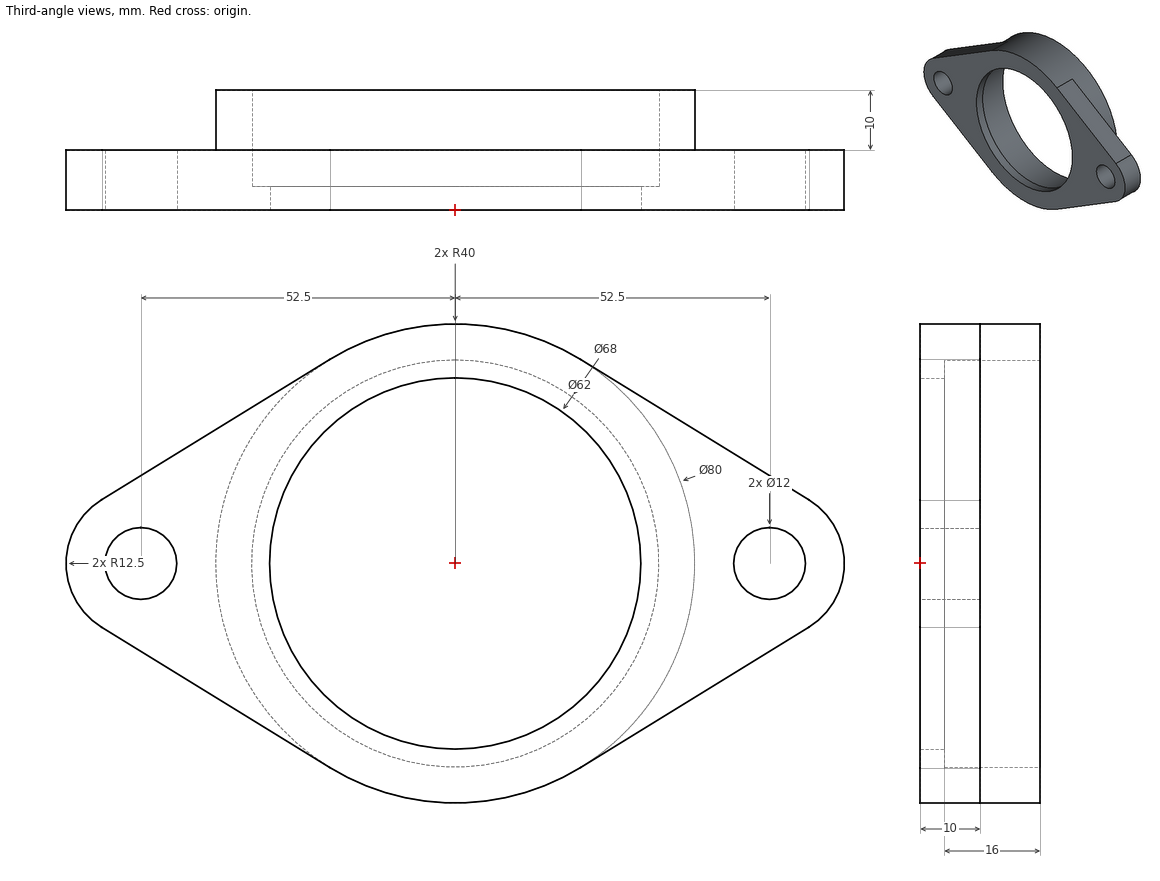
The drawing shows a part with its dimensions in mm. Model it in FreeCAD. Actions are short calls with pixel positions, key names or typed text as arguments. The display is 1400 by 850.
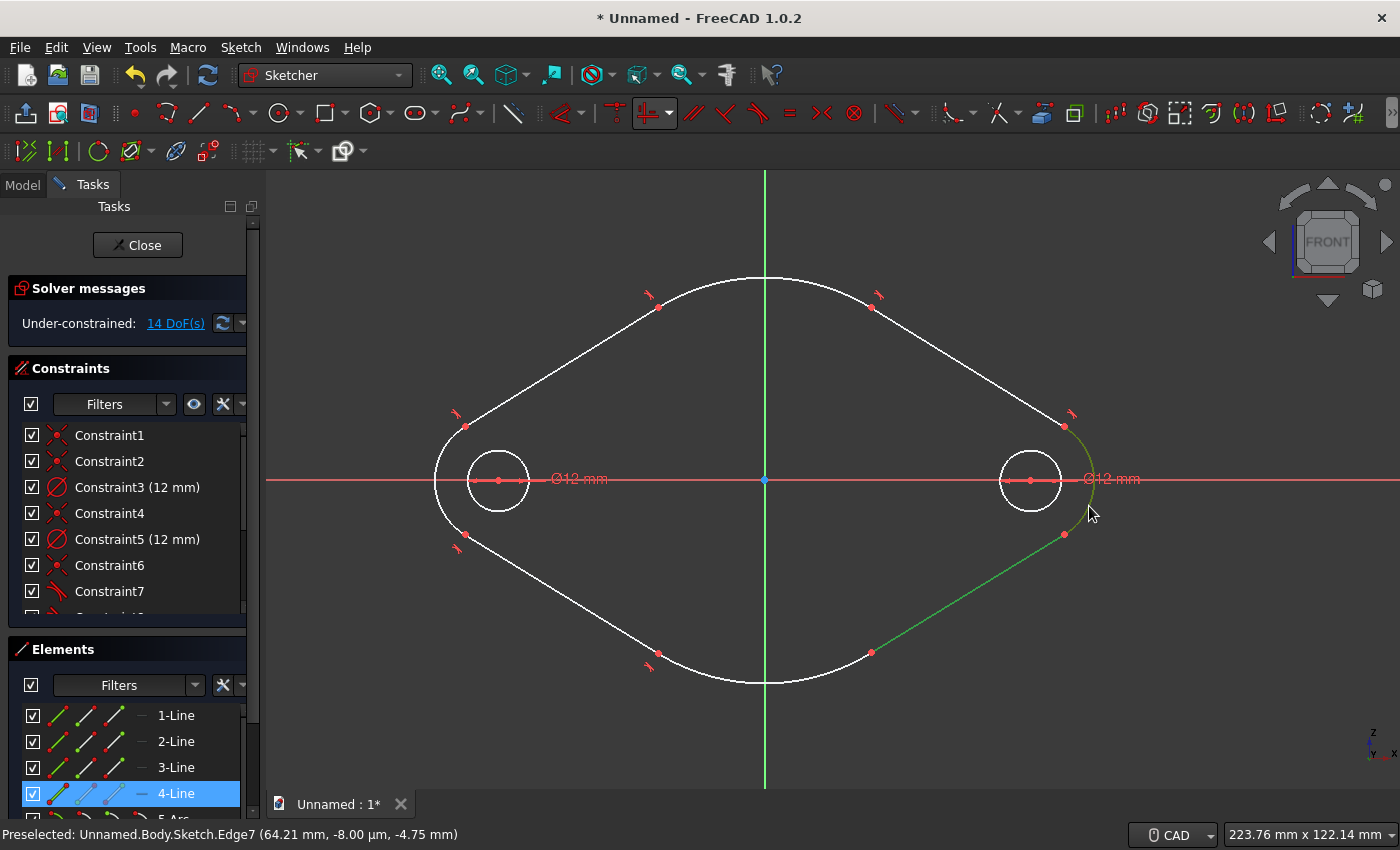
click(758, 114)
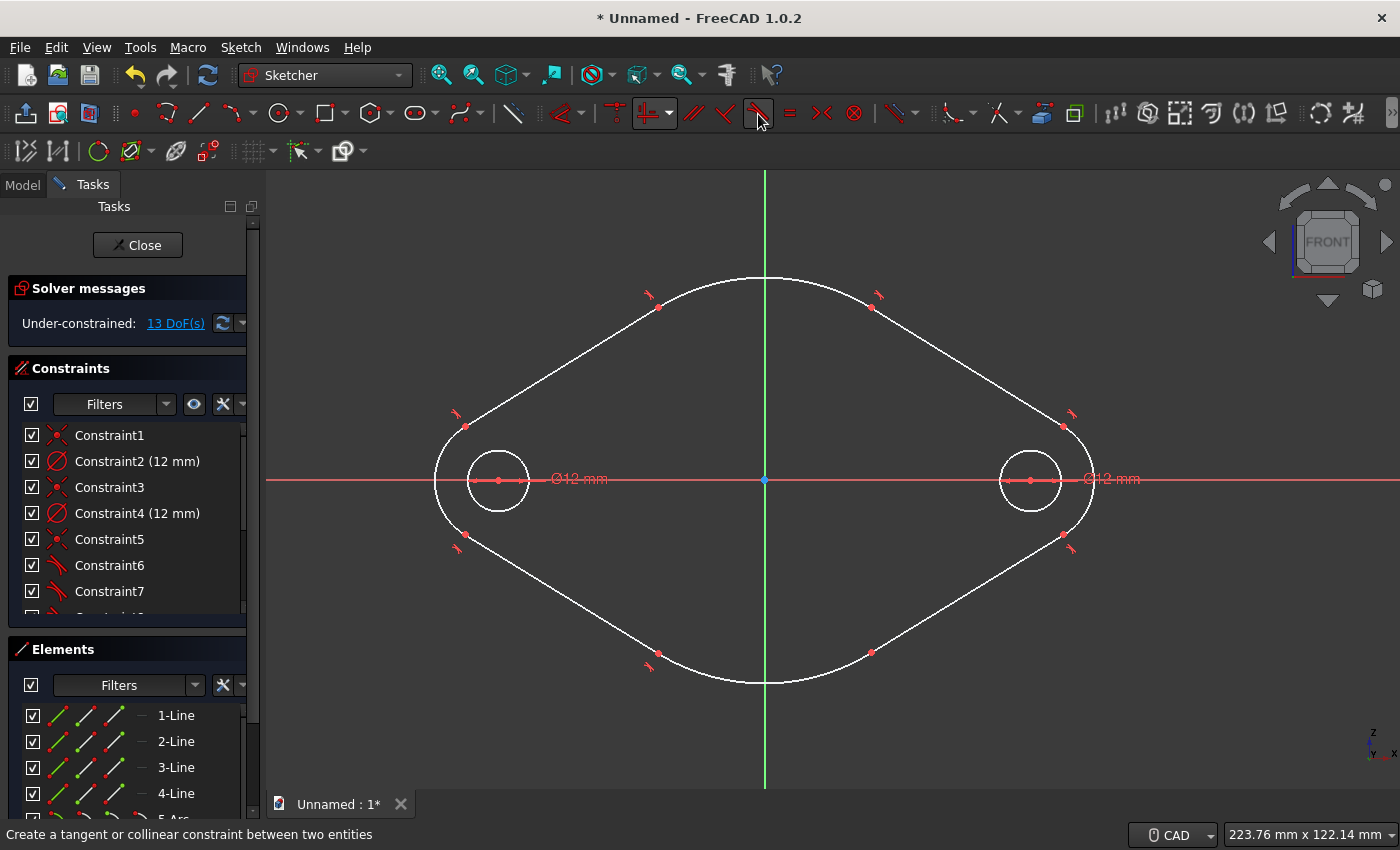
click(1006, 570)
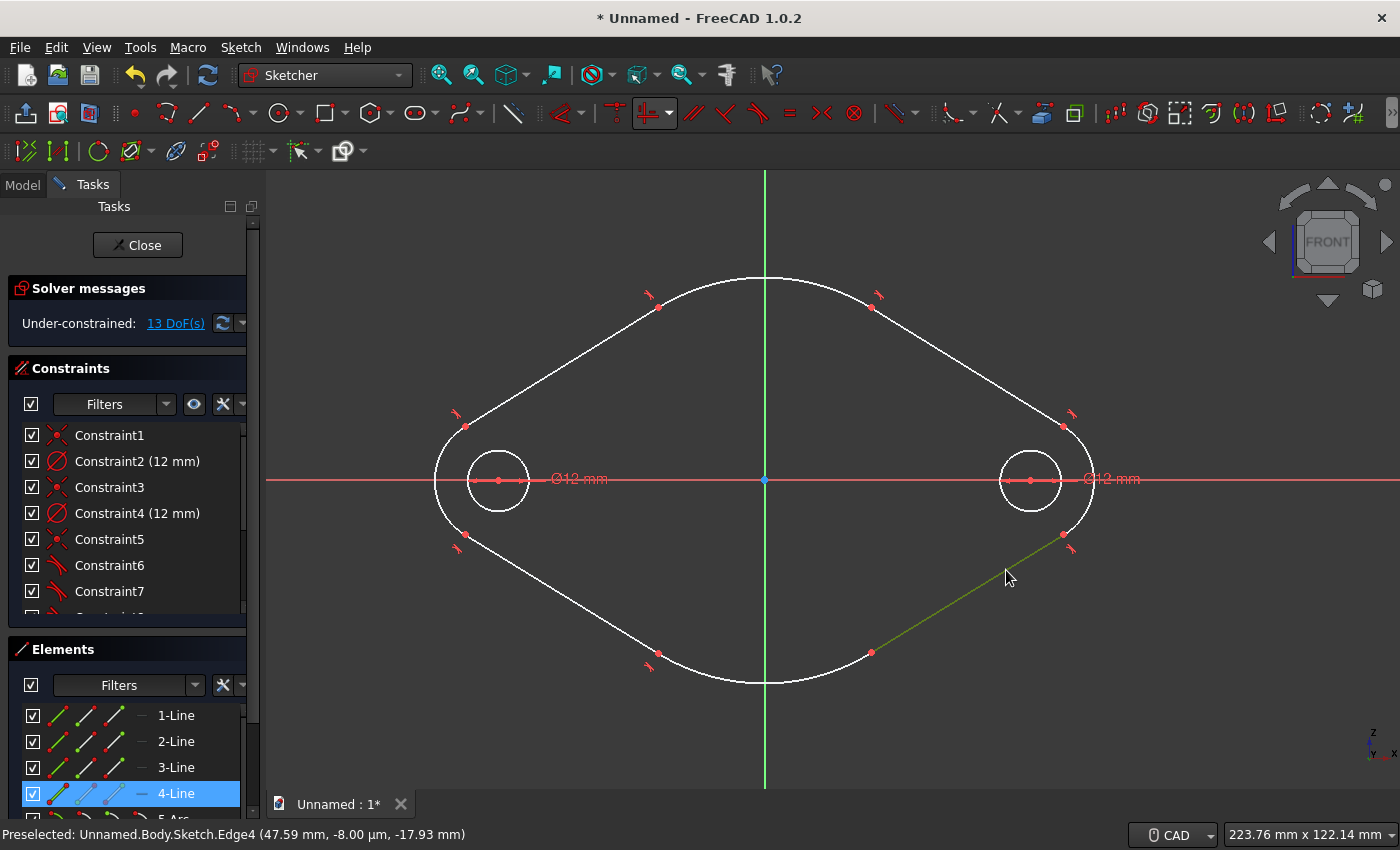
click(720, 679)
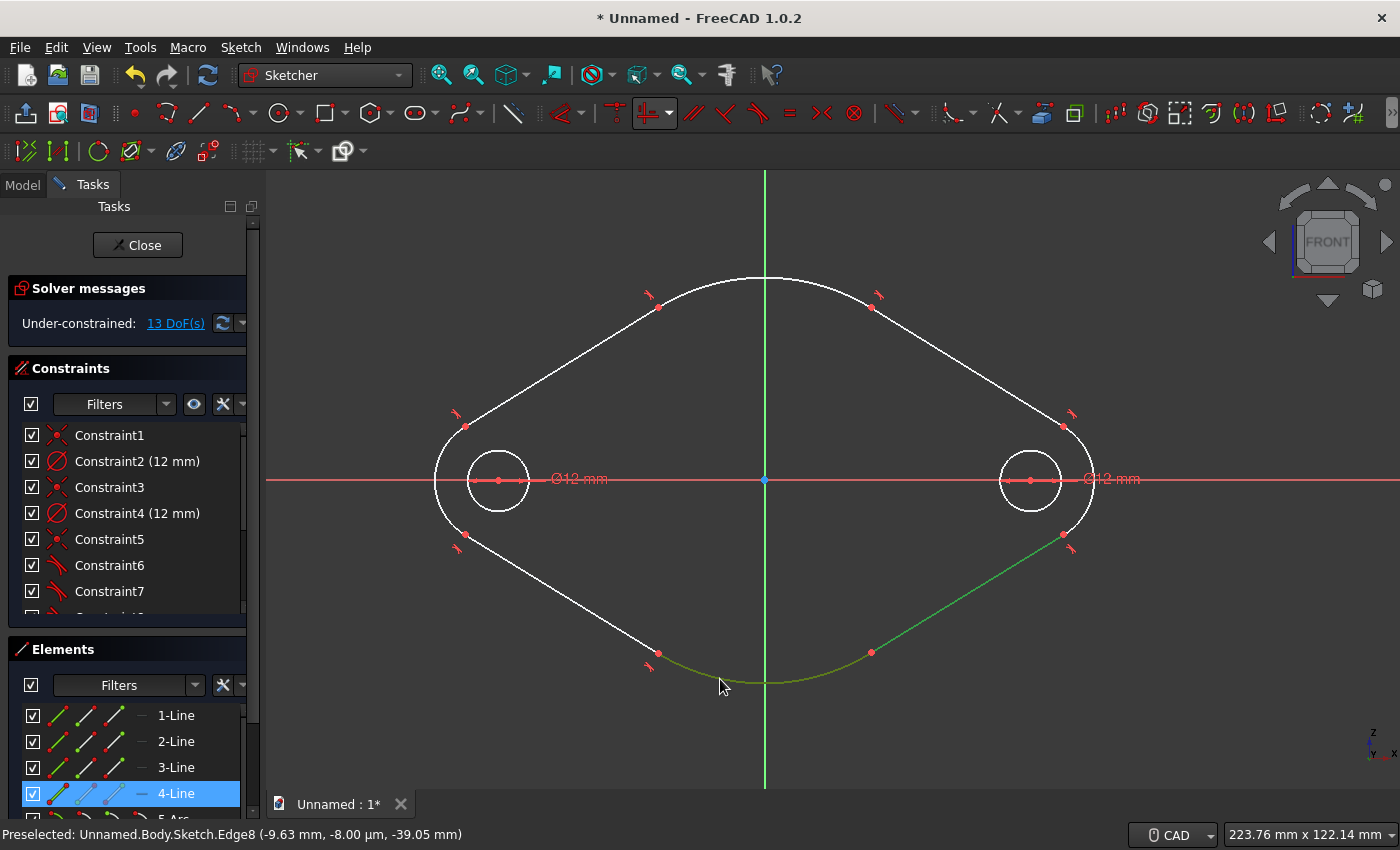
click(758, 114)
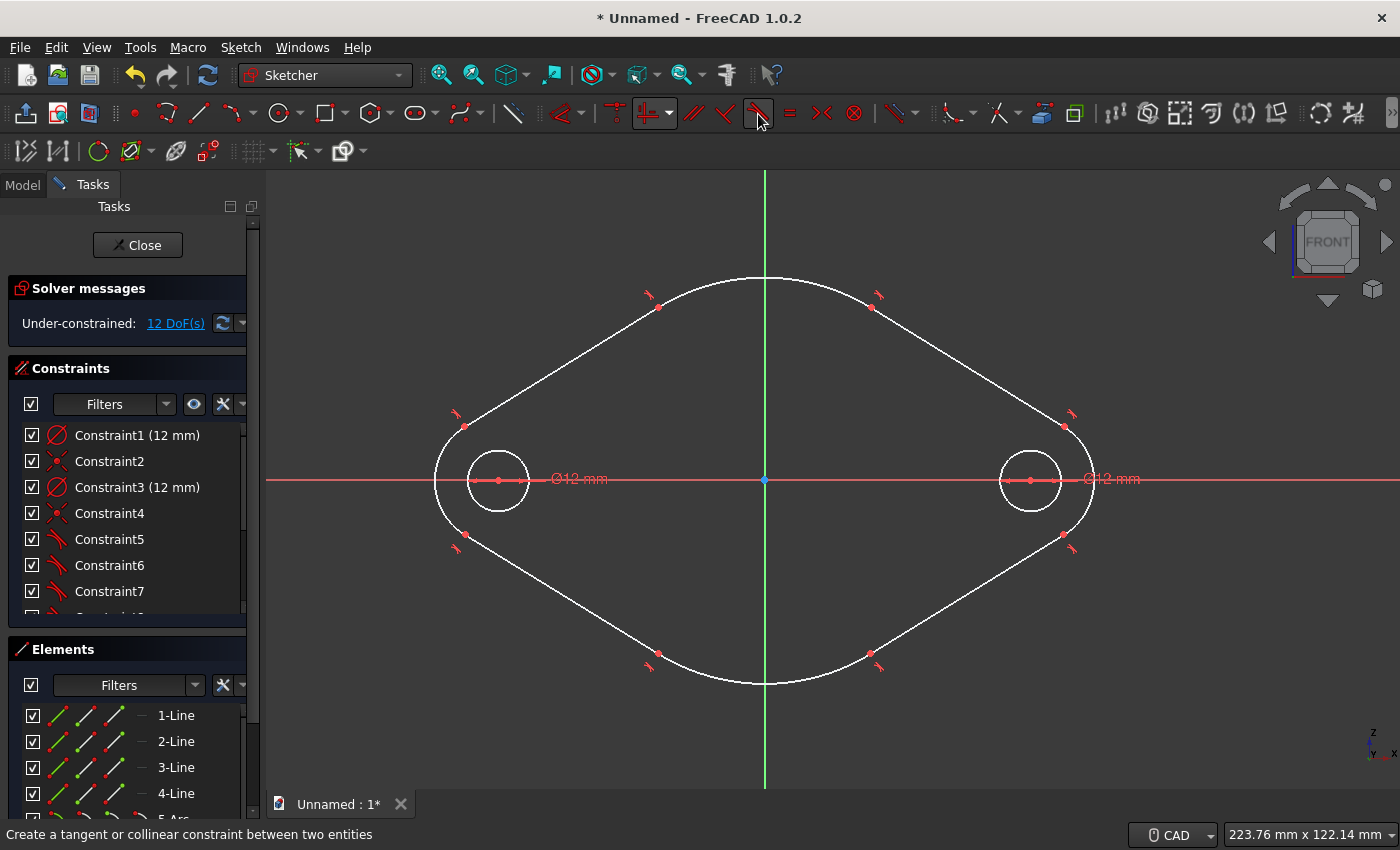
click(809, 283)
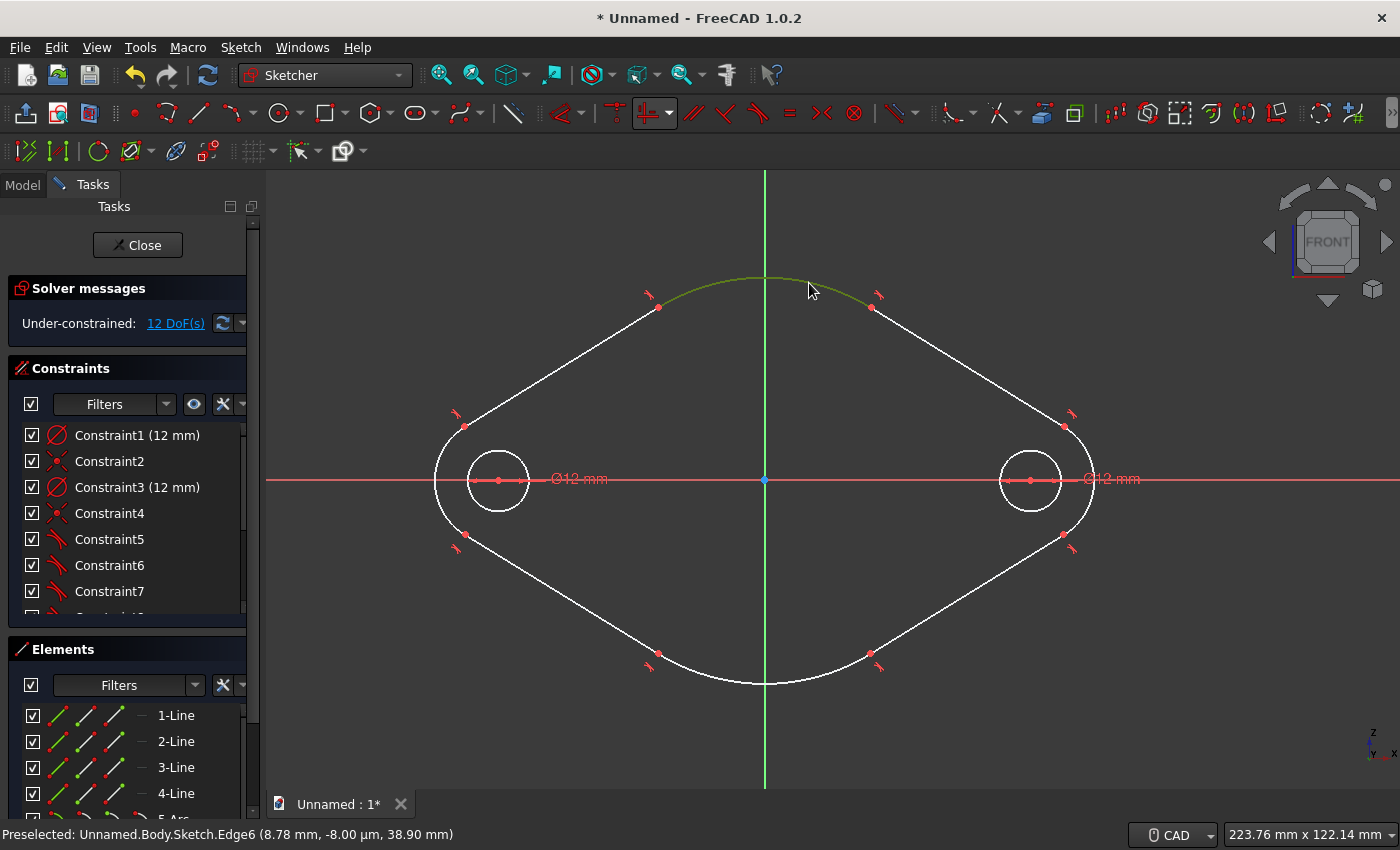
click(720, 679)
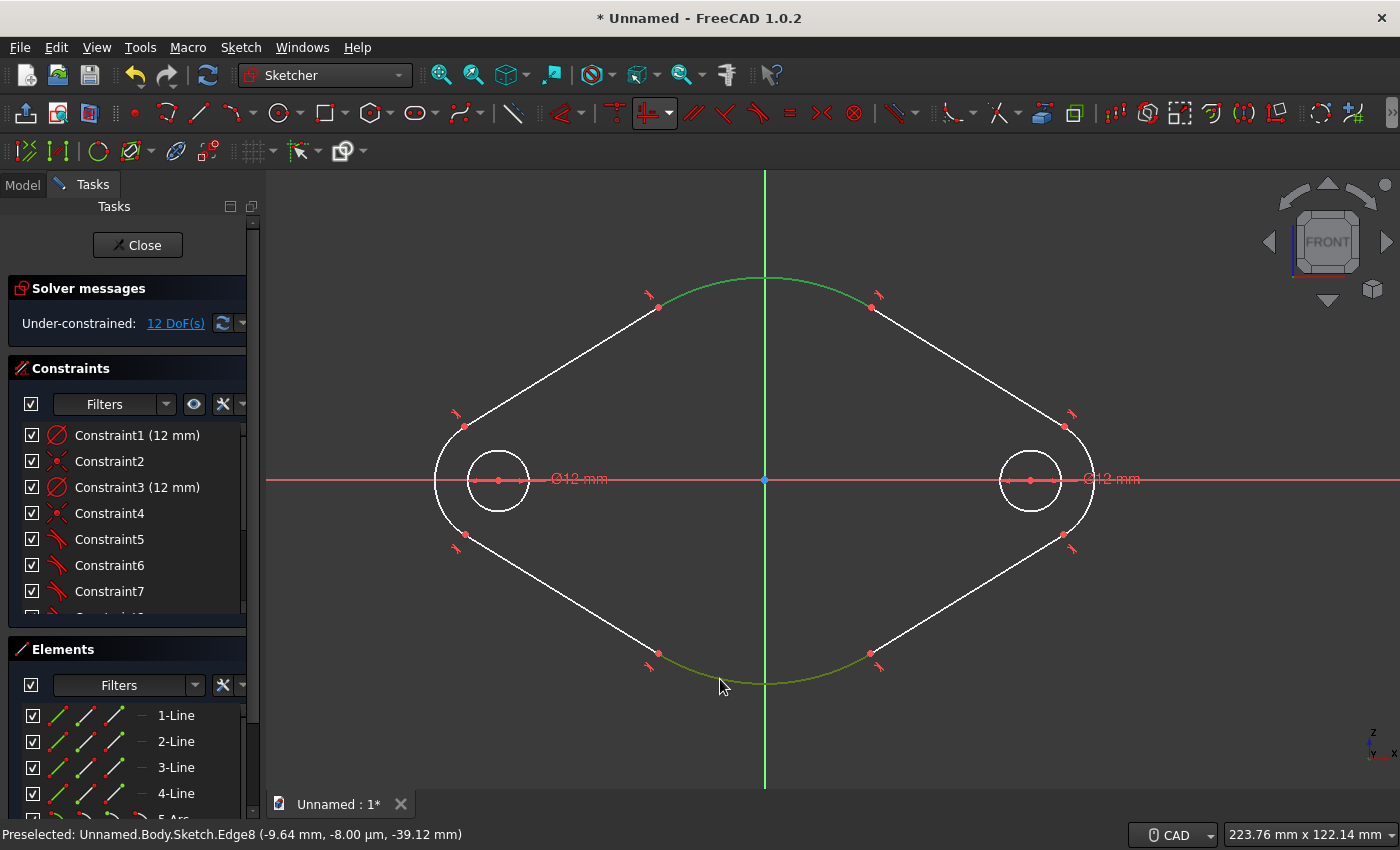
click(616, 114)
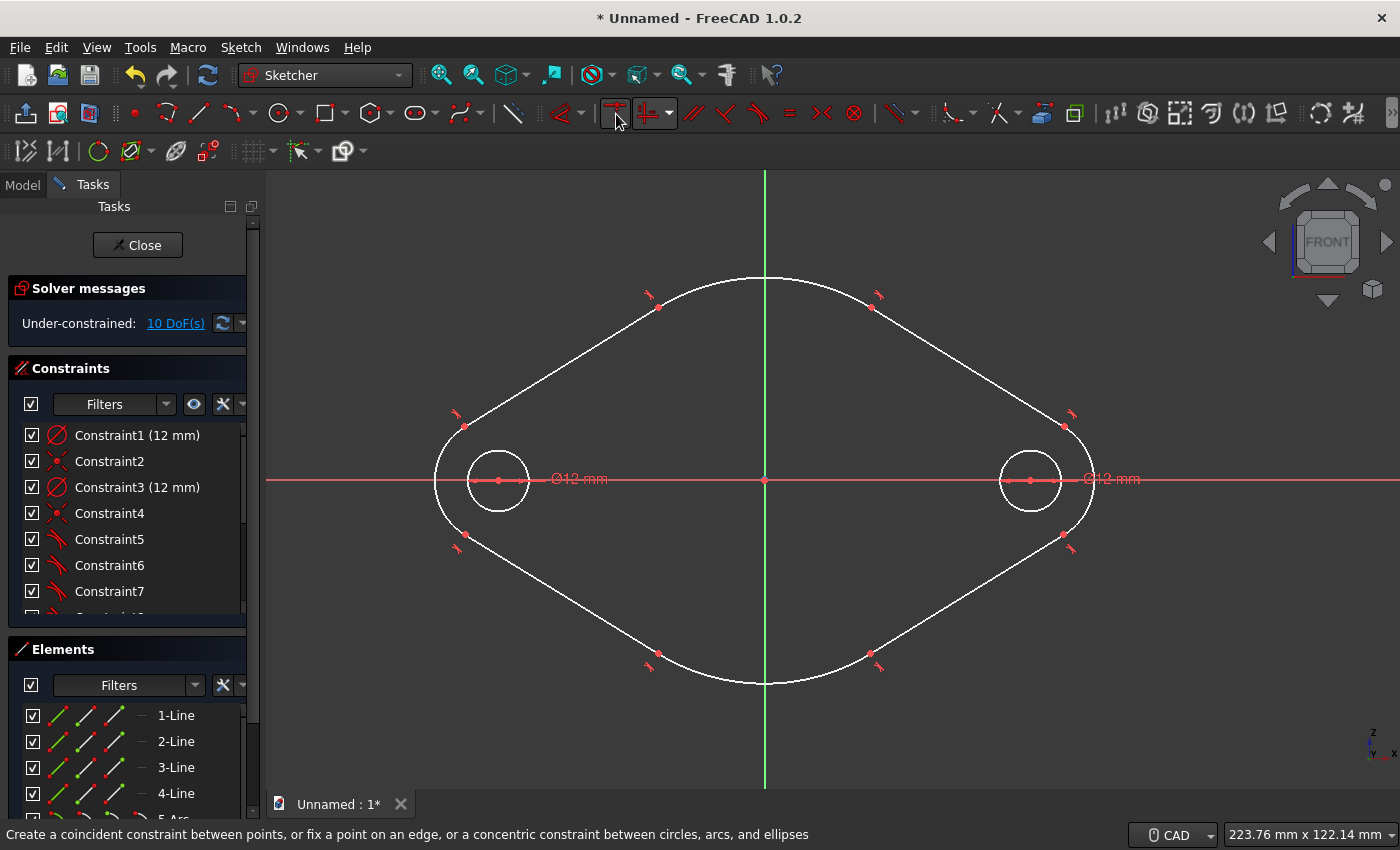
scroll(765, 480, up, 2)